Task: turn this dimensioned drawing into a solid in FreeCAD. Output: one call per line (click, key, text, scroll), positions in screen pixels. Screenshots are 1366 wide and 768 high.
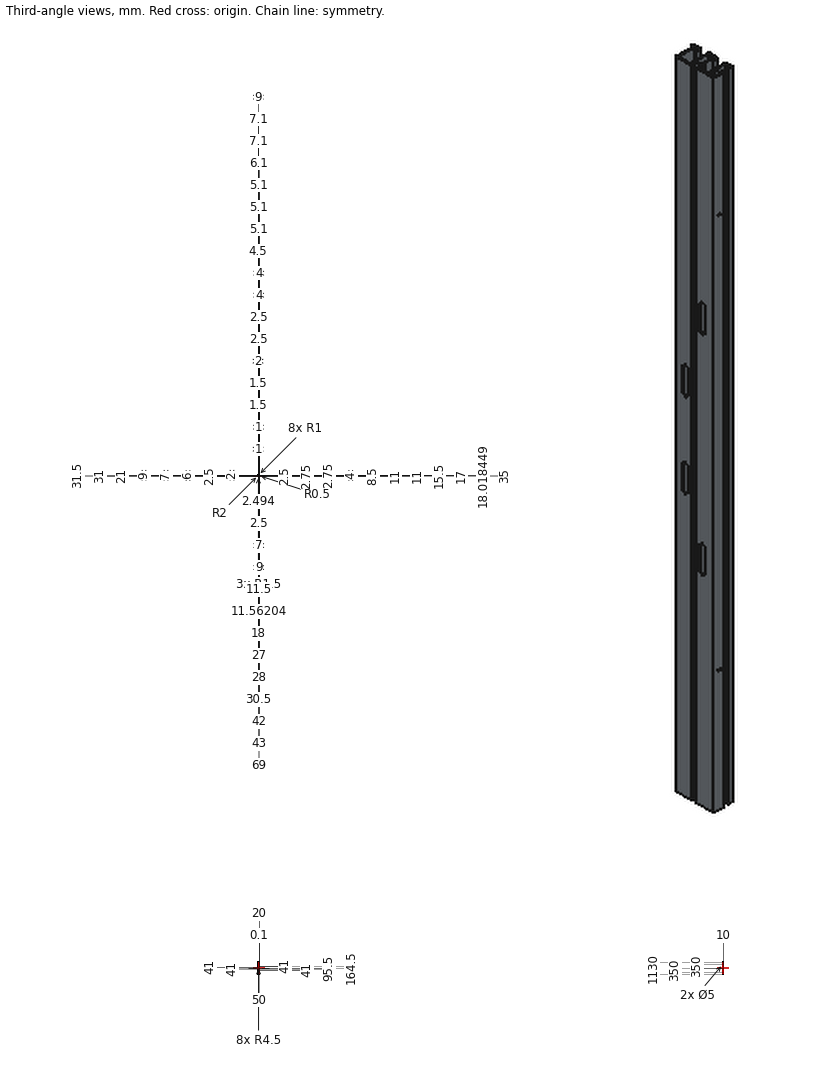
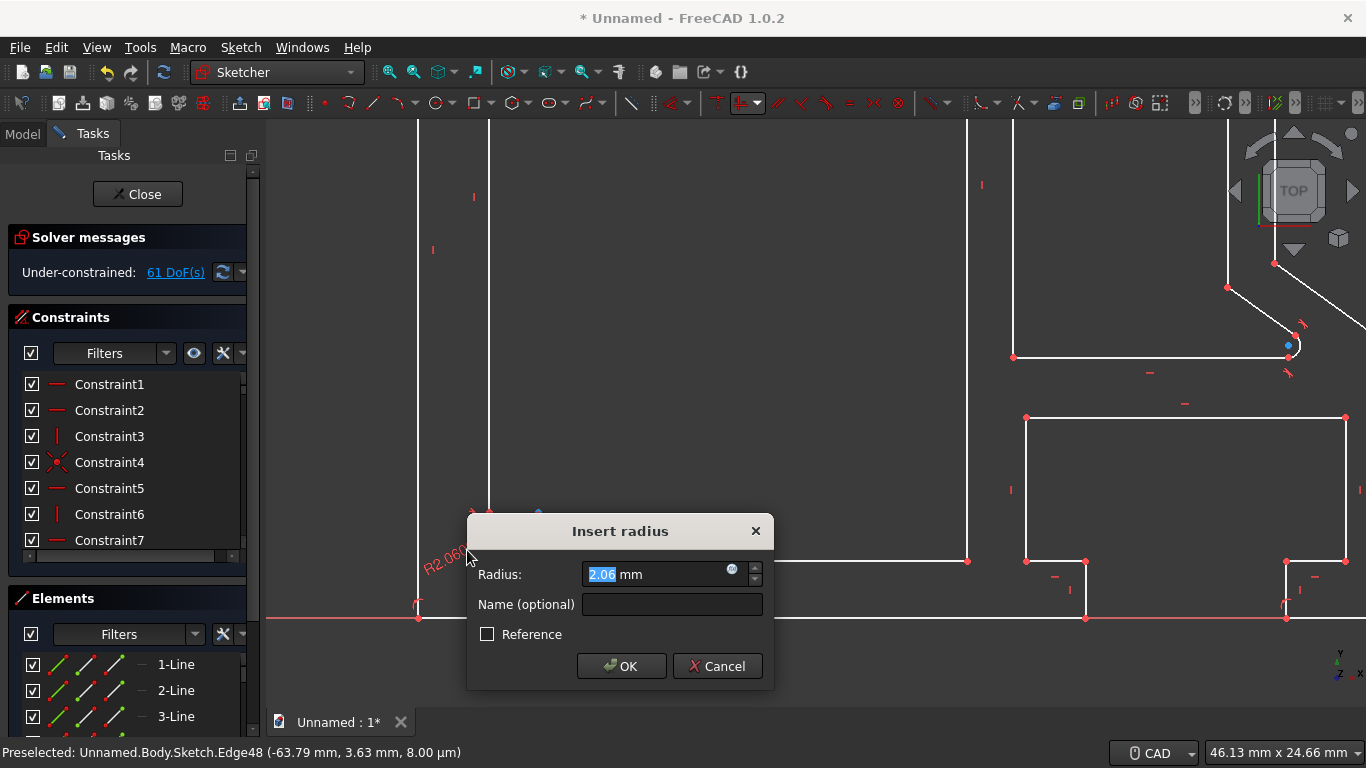
text(2)
key(Return)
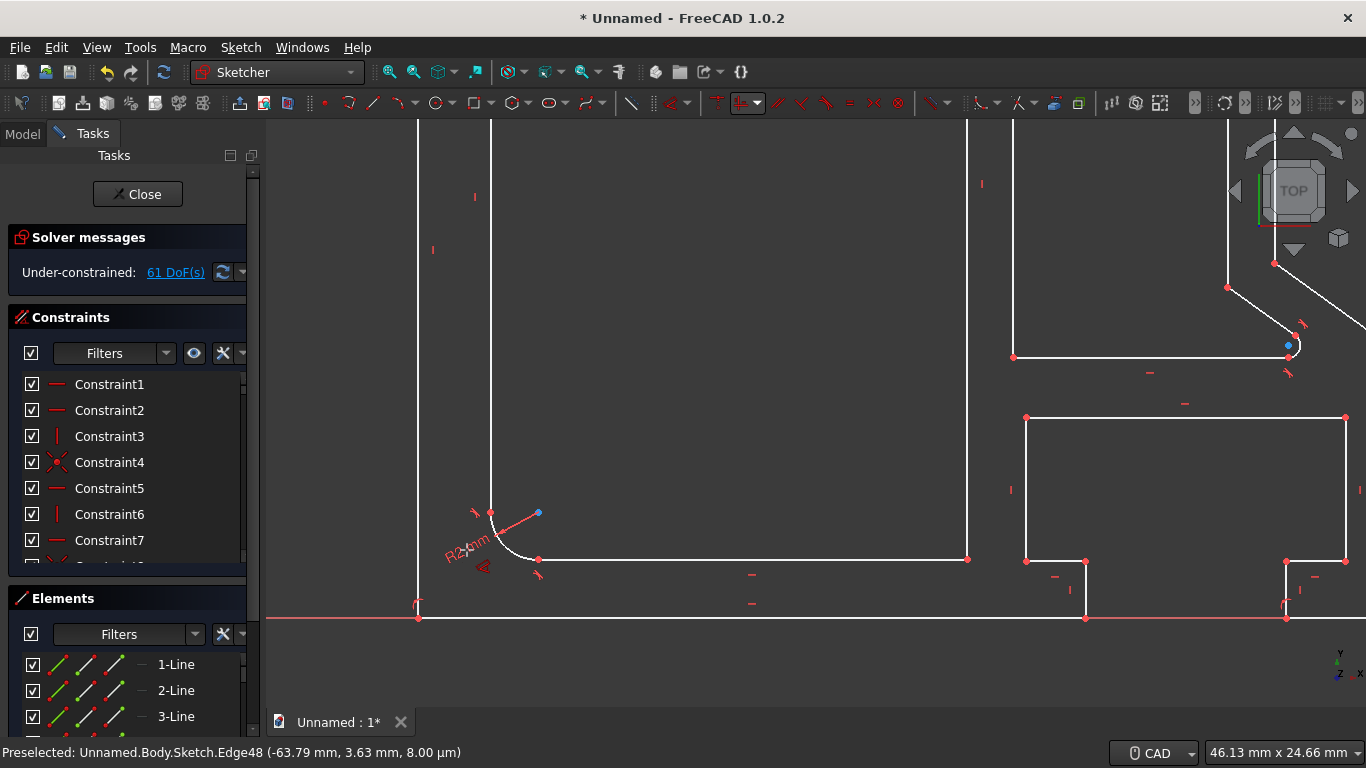
scroll(496, 536, down, 5)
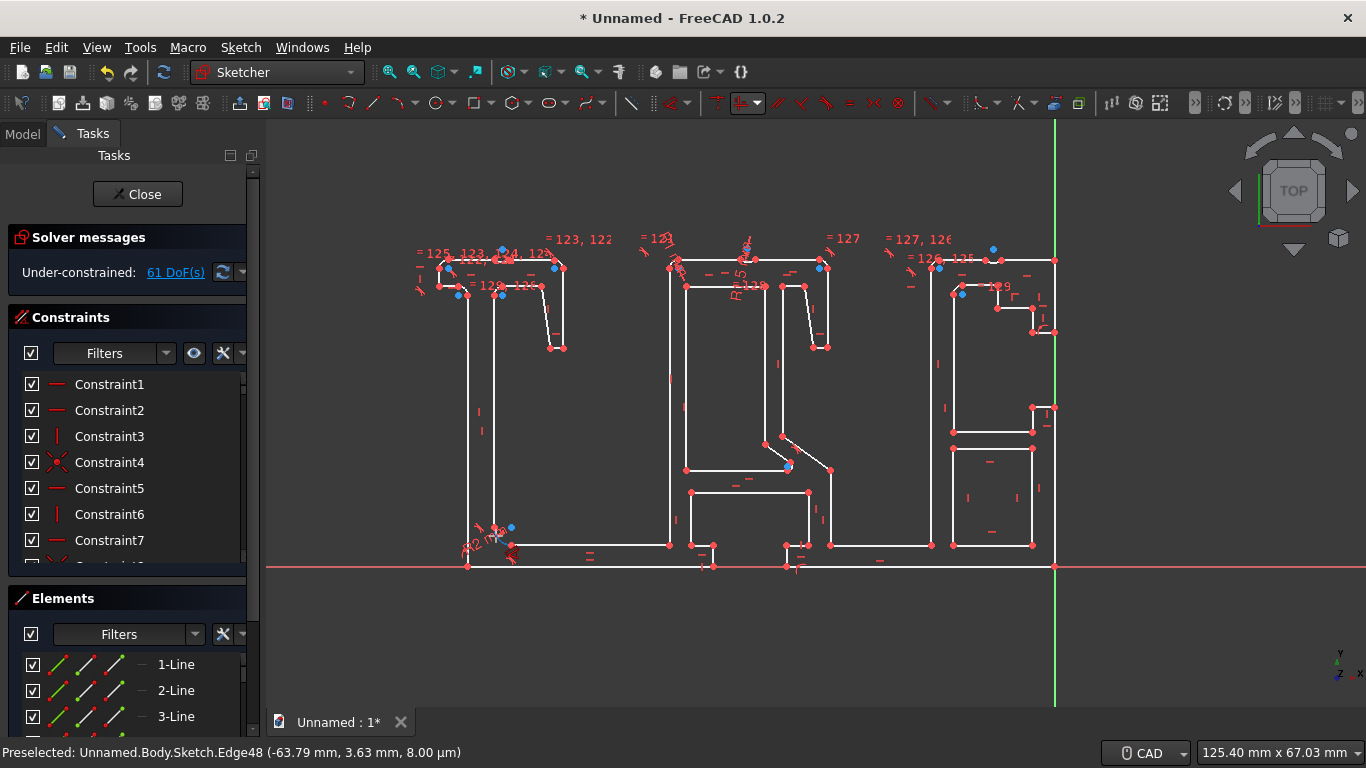
scroll(791, 470, up, 12)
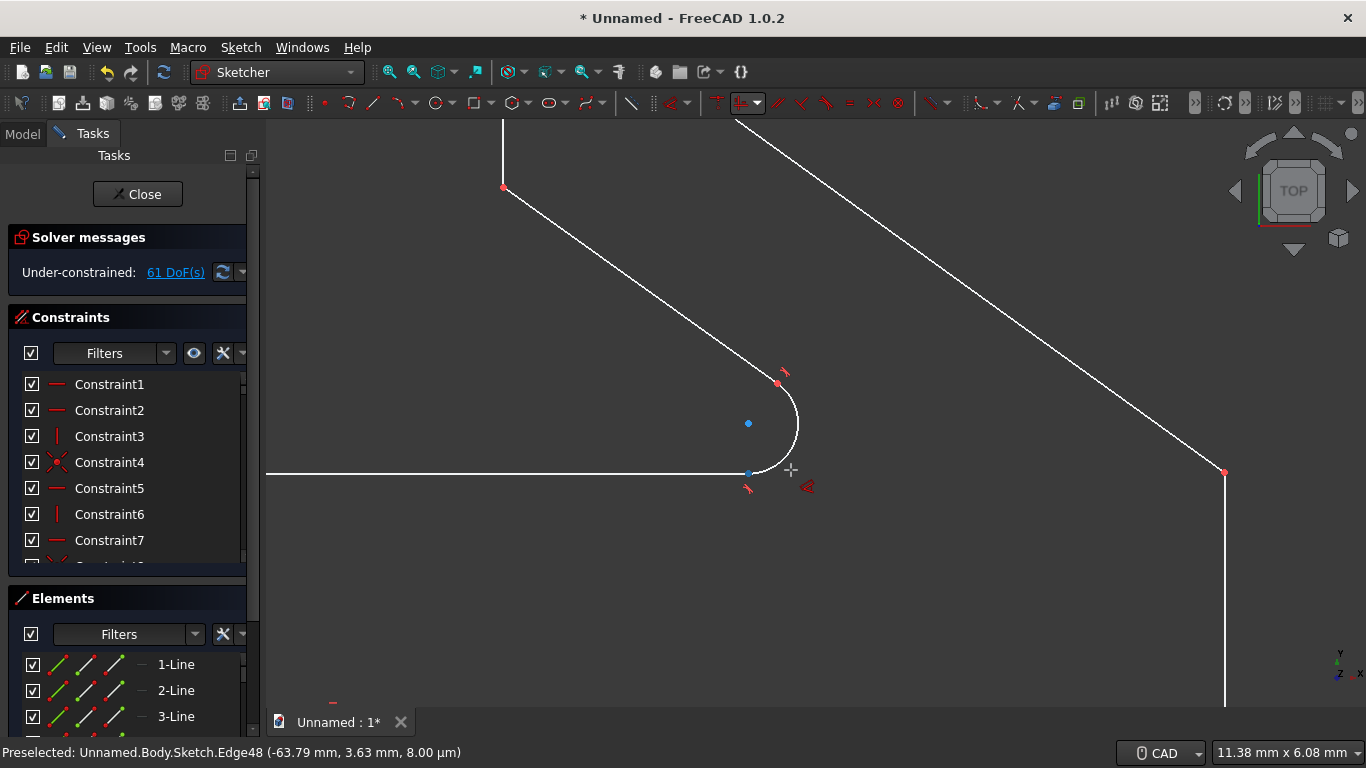
click(782, 460)
click(804, 483)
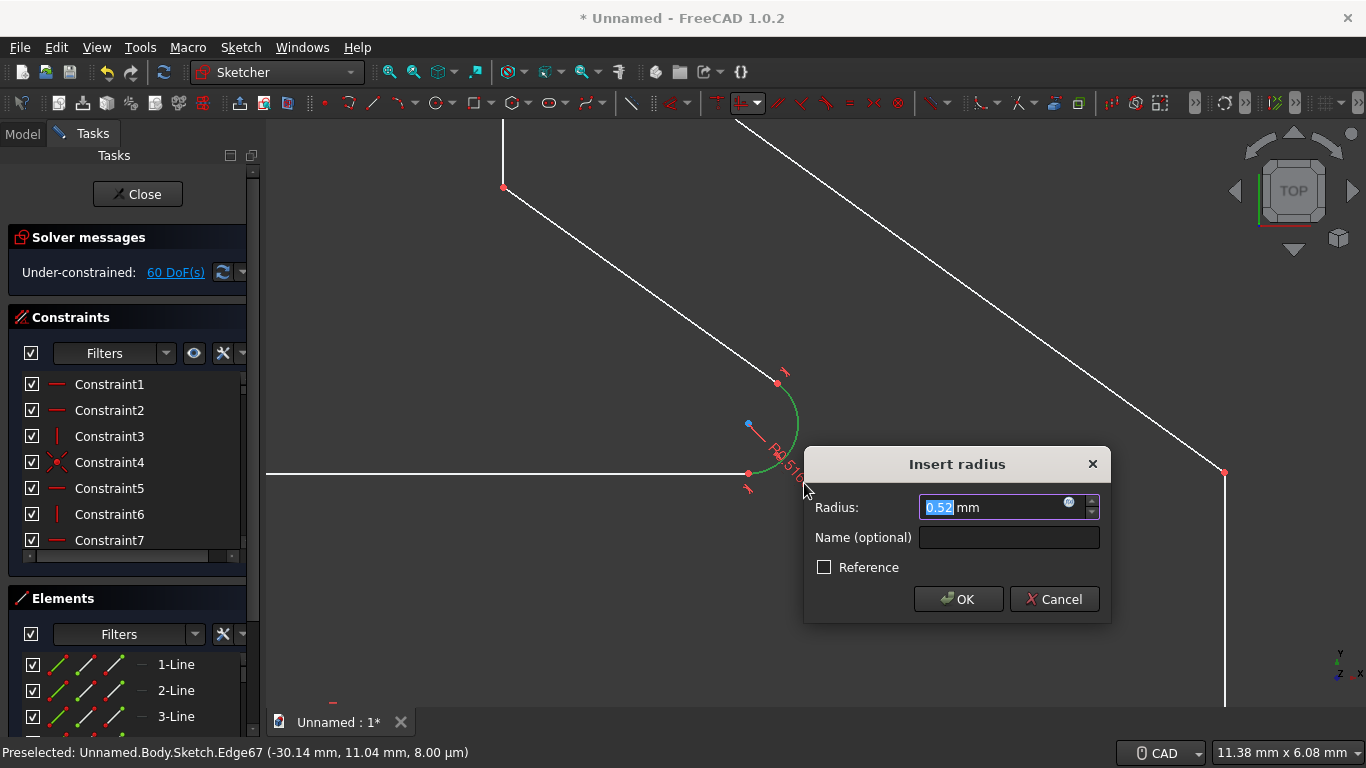
text(0.5)
key(Return)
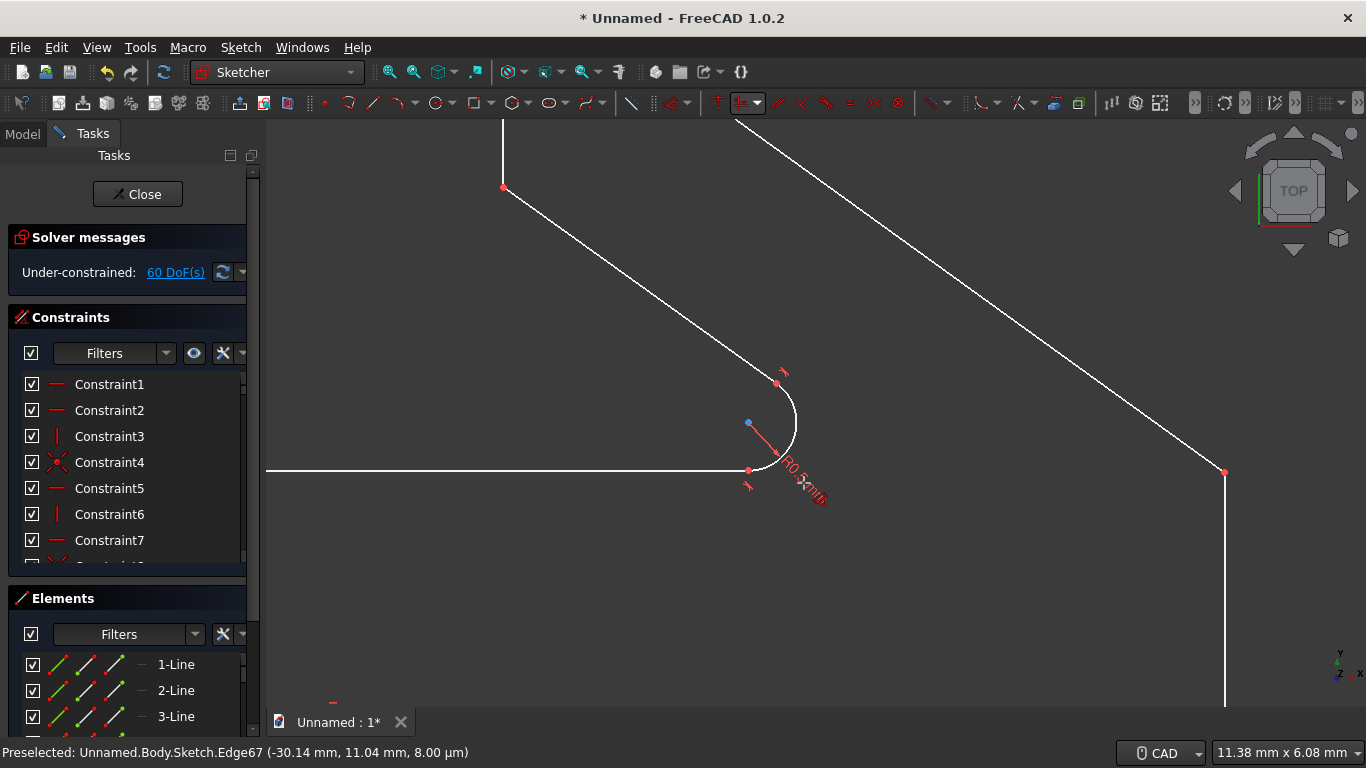
scroll(791, 470, down, 12)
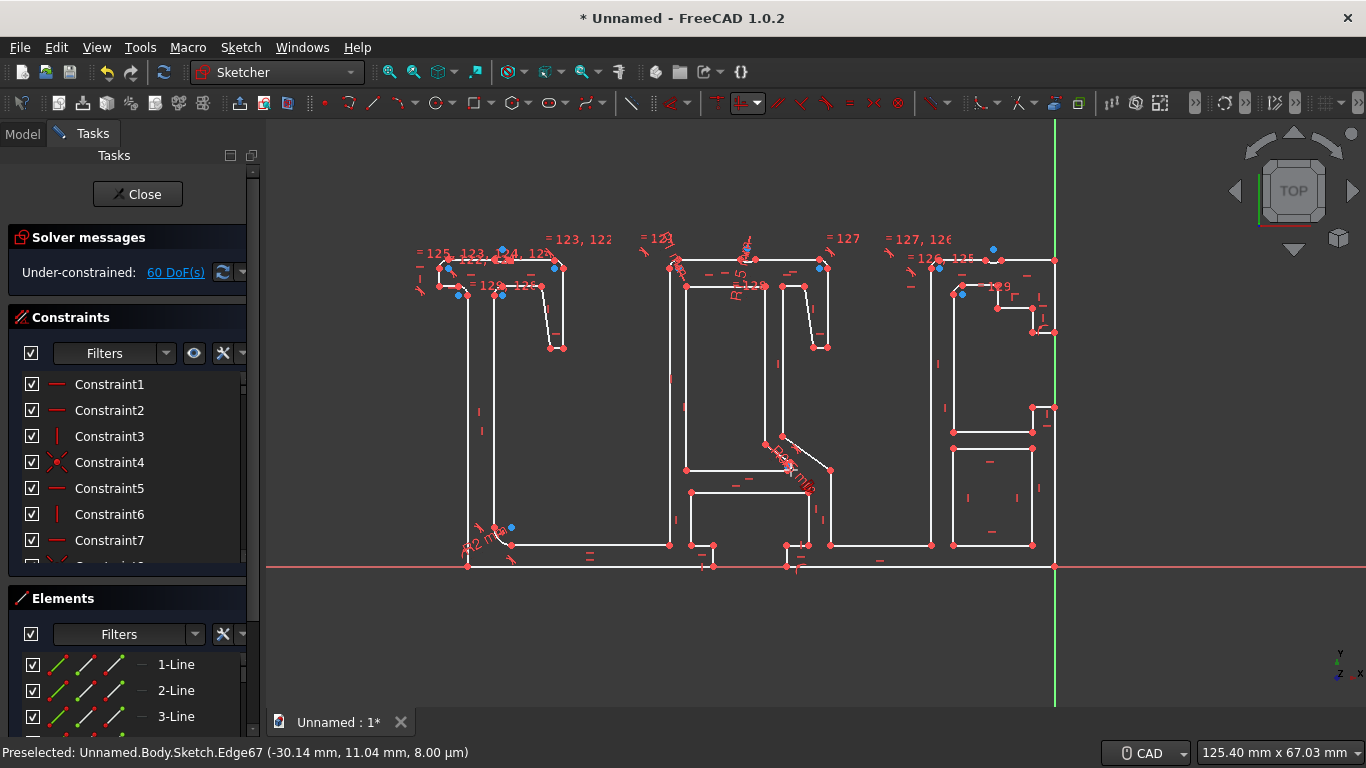
click(563, 324)
click(529, 309)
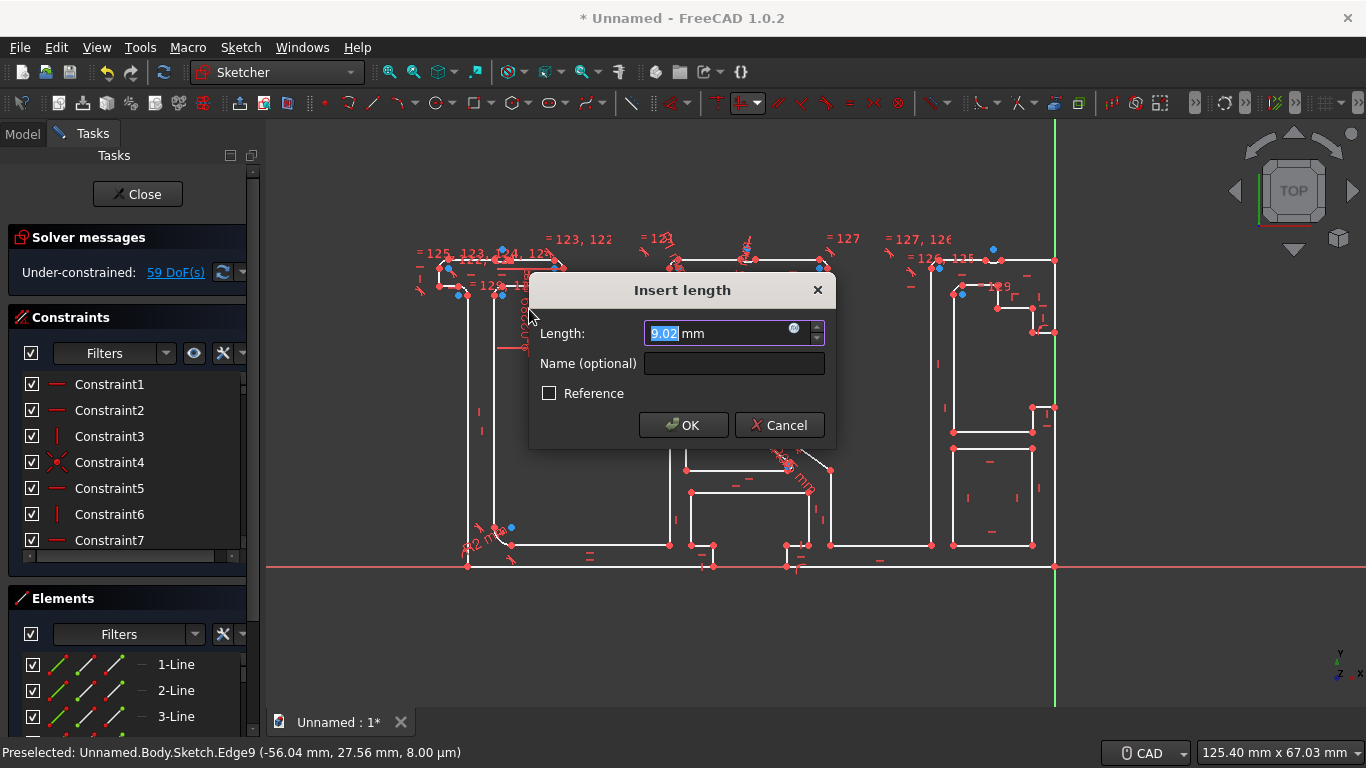
text(9)
key(Return)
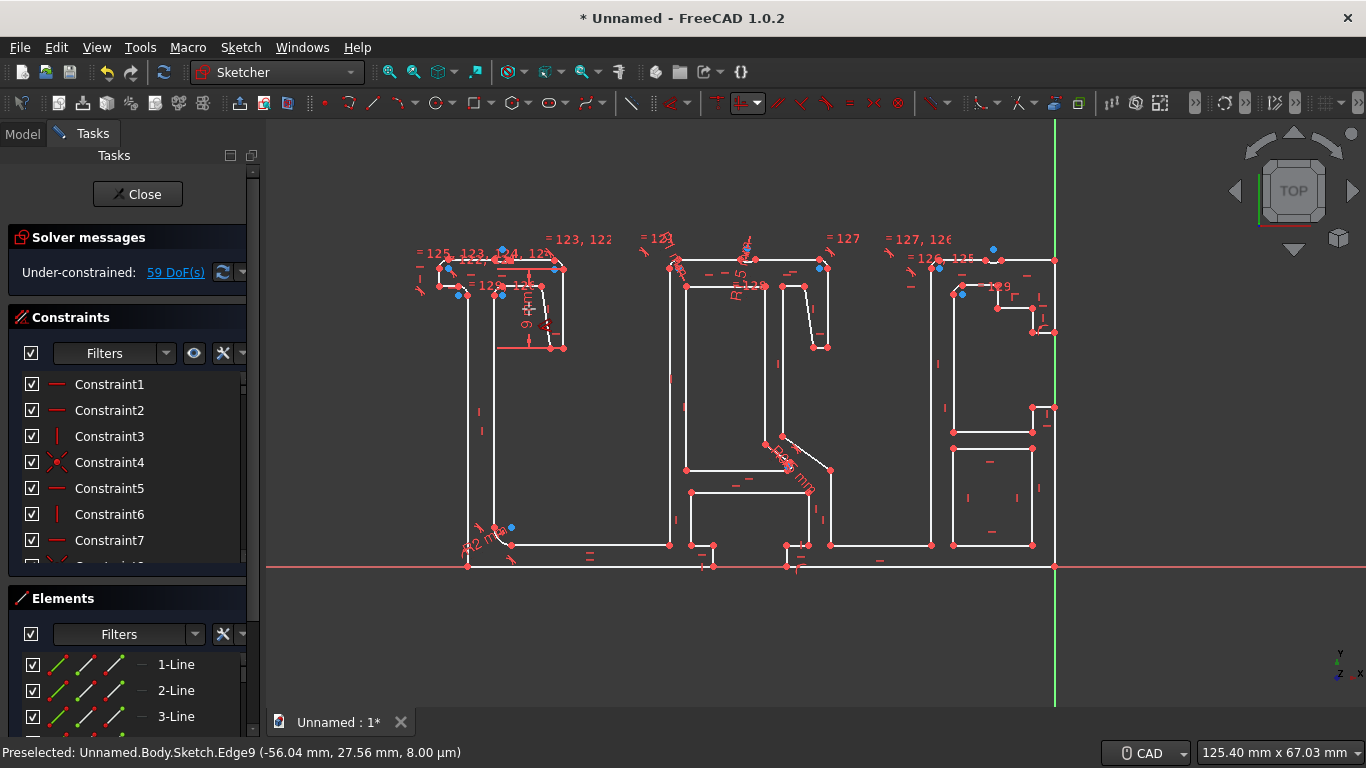
scroll(439, 277, up, 5)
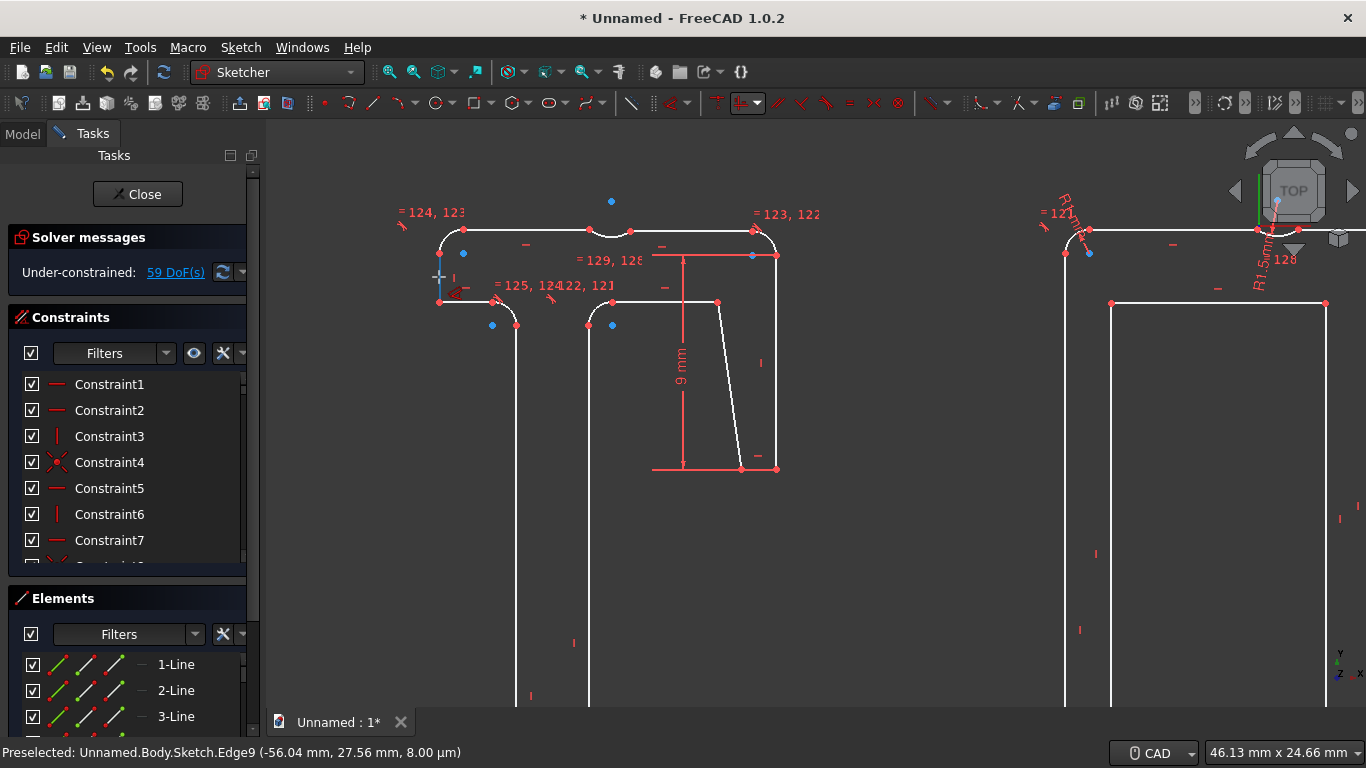
click(440, 278)
click(406, 278)